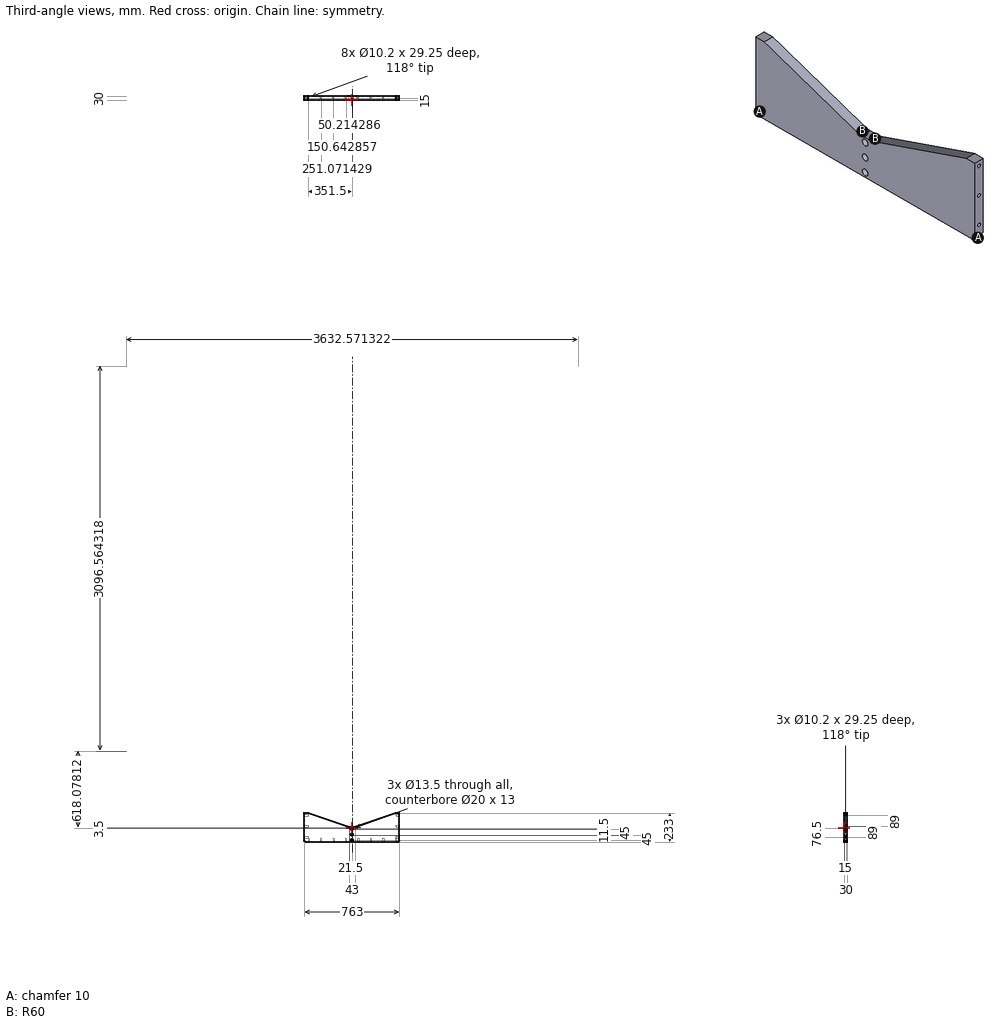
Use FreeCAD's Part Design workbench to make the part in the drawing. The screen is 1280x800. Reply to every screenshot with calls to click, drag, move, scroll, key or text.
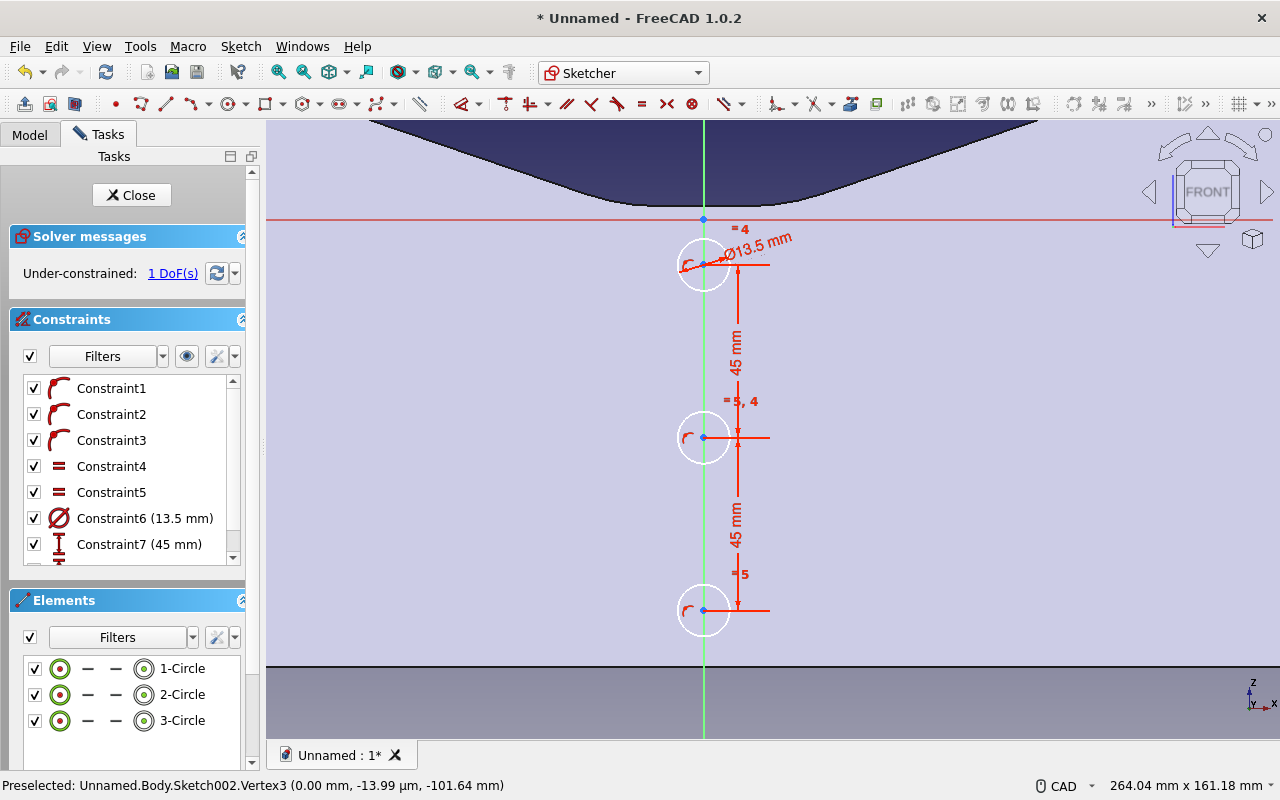
click(704, 265)
click(670, 242)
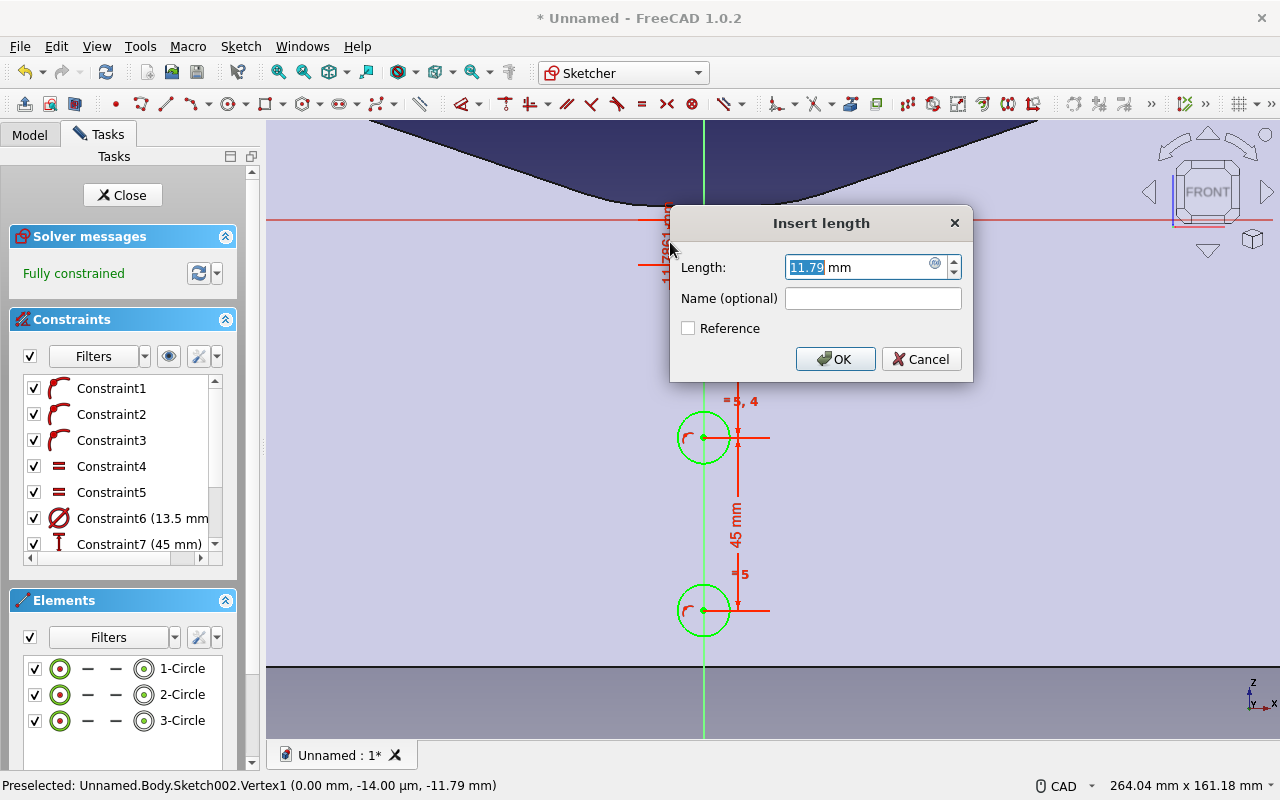
text(11.5)
key(Return)
key(Escape)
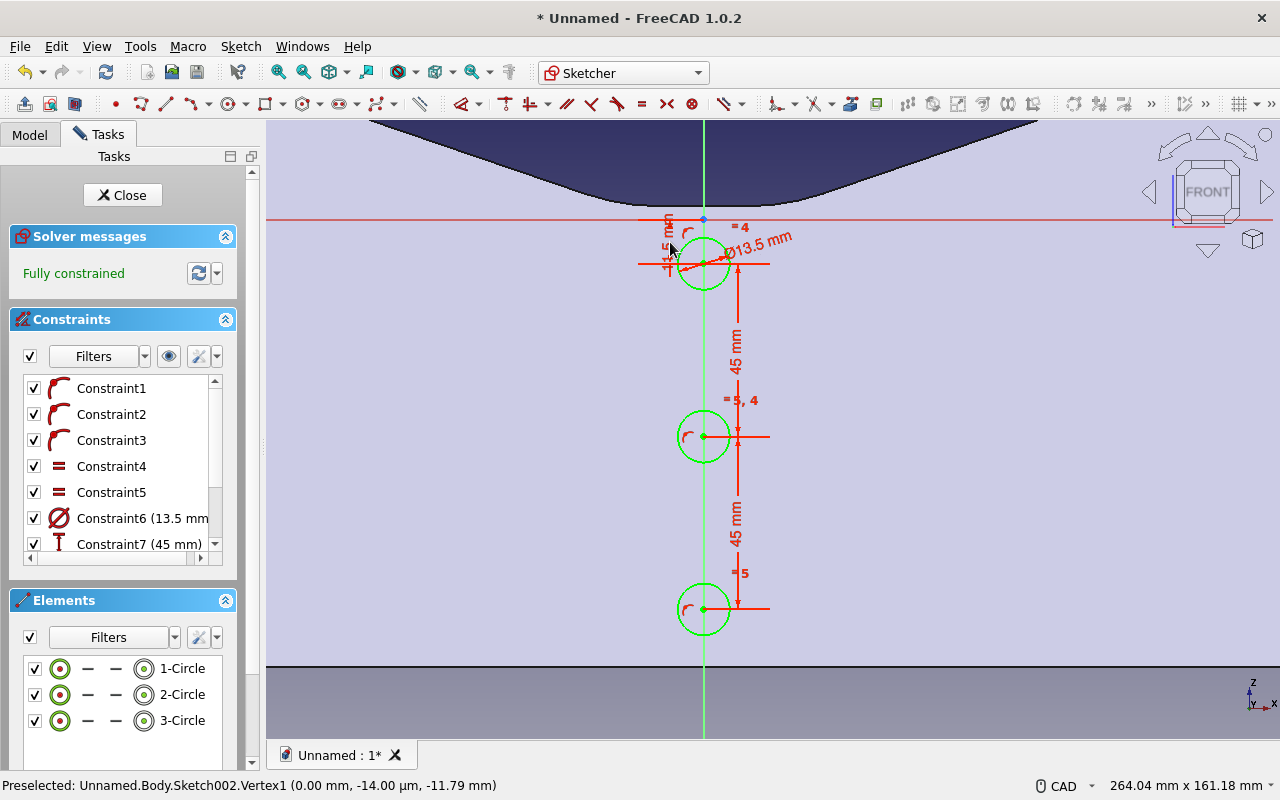
click(123, 195)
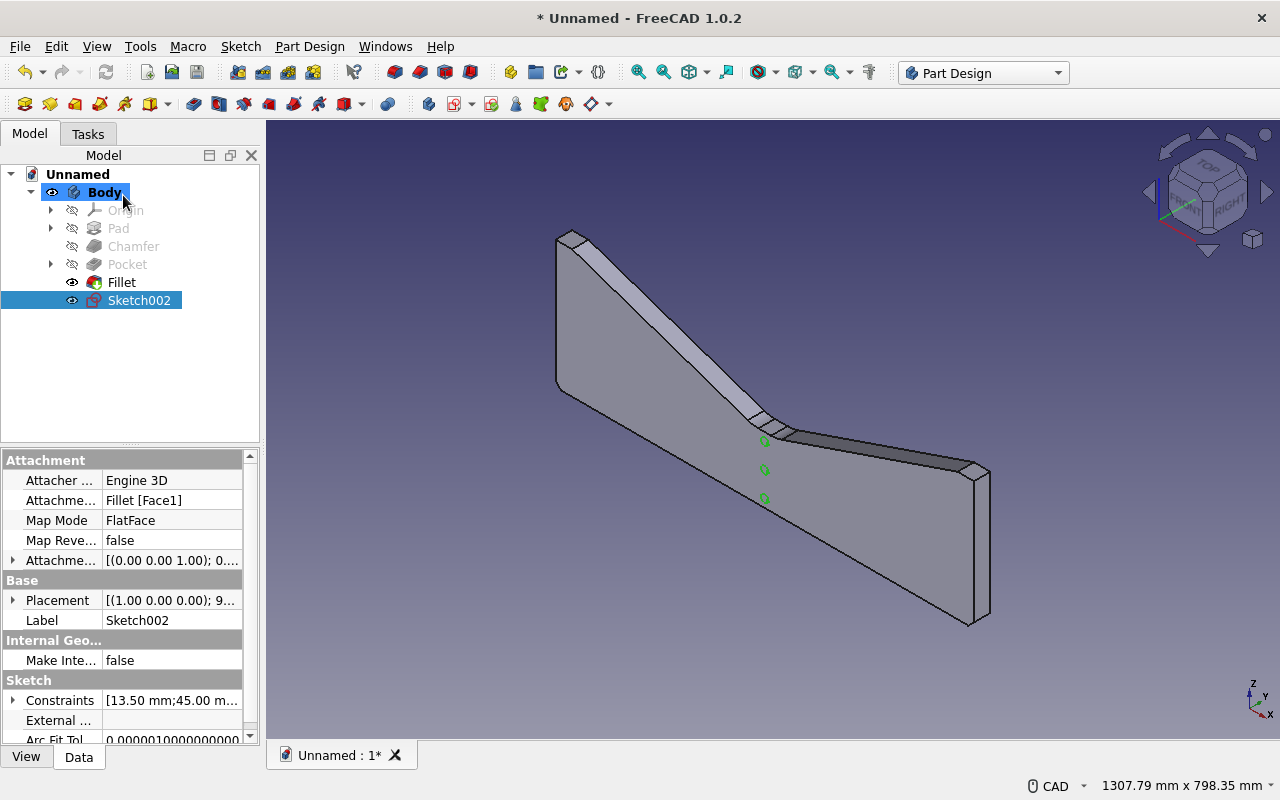
click(219, 104)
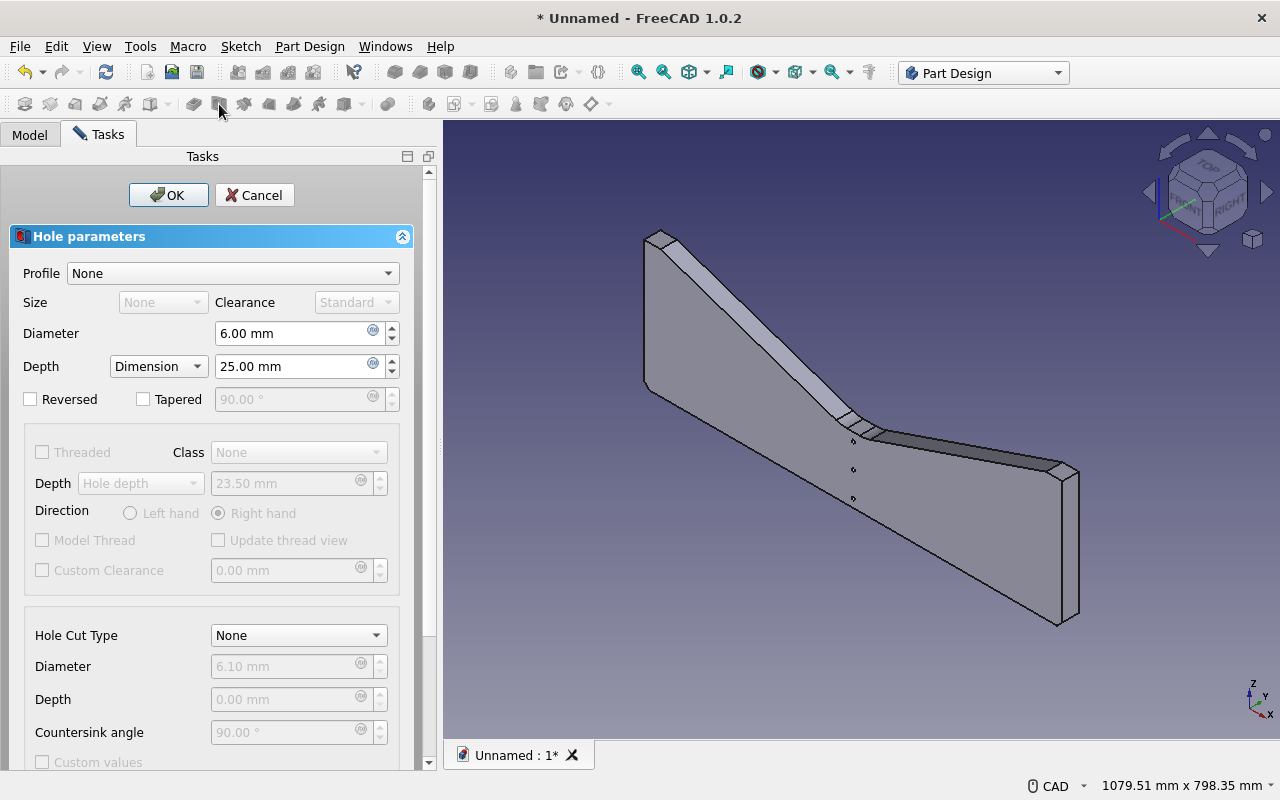
triple_click(300, 334)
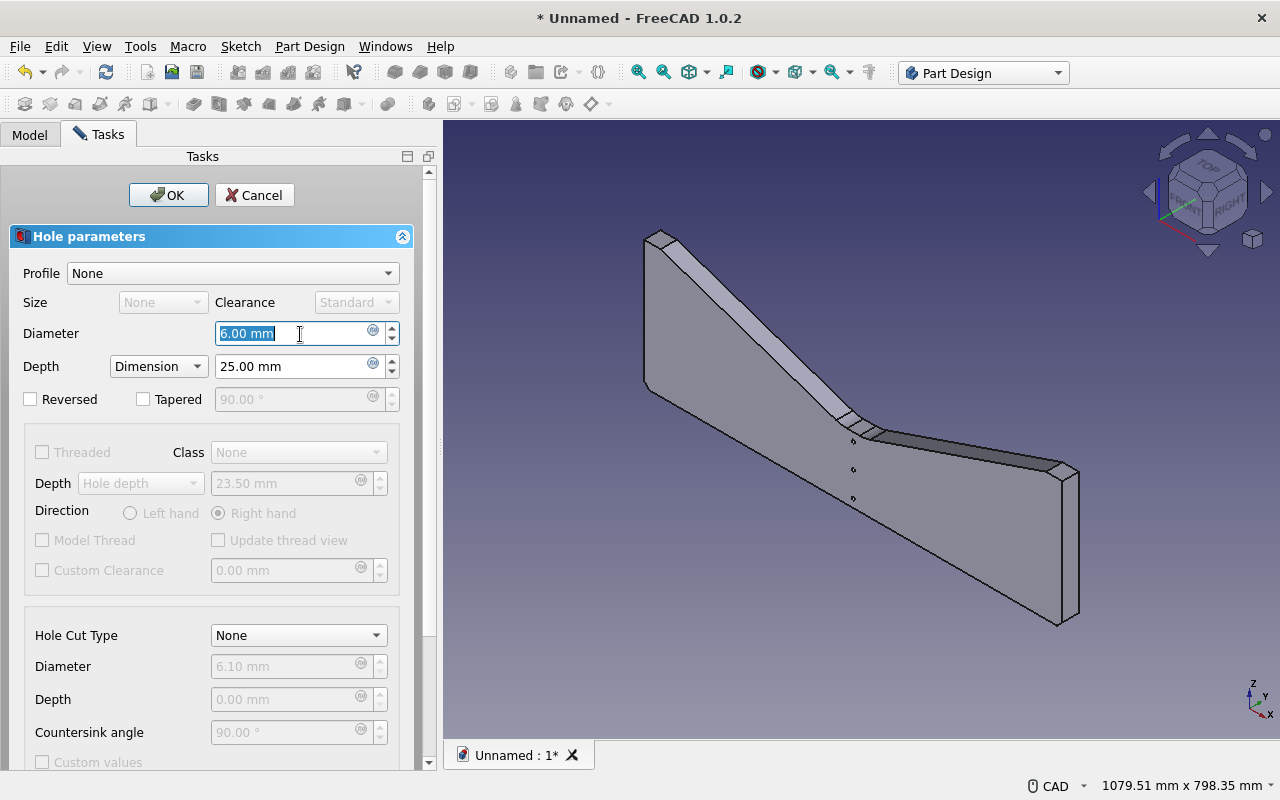
text(13.5)
key(Tab)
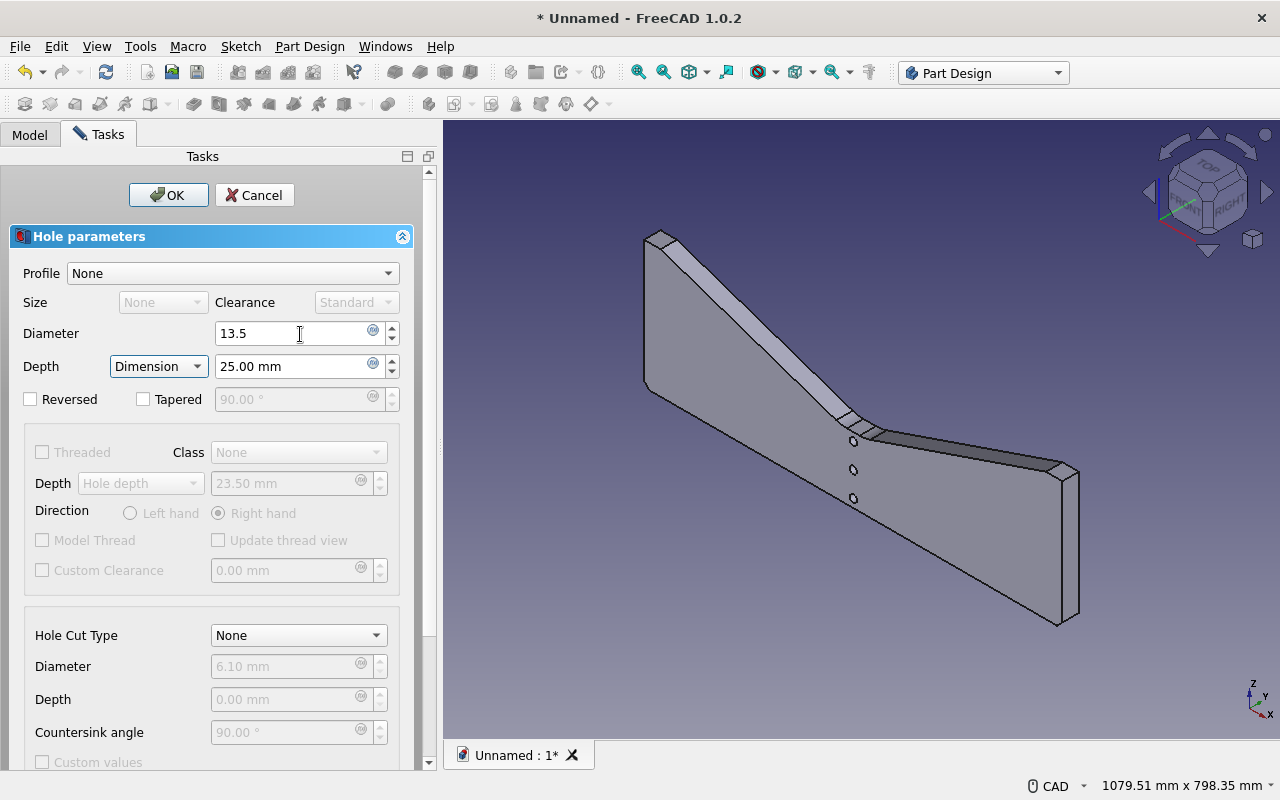
click(160, 366)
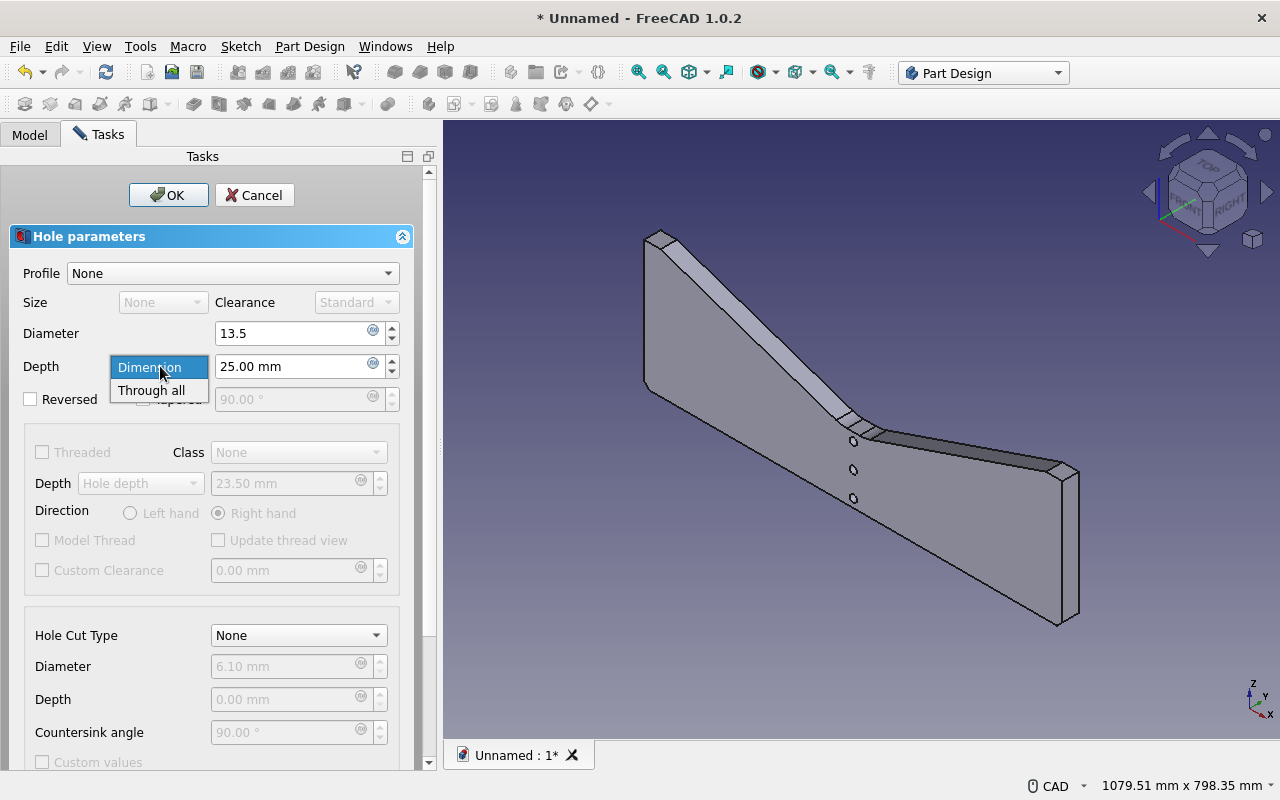
click(158, 390)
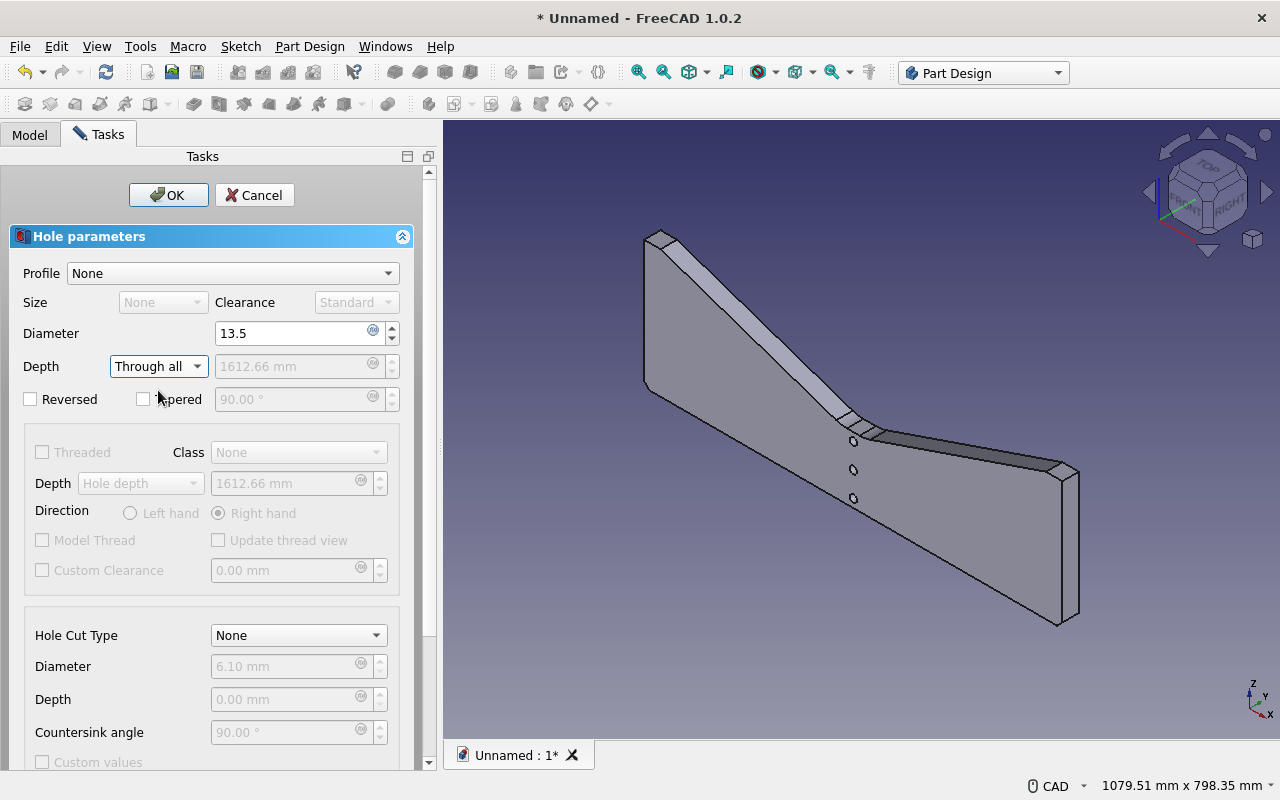
click(300, 636)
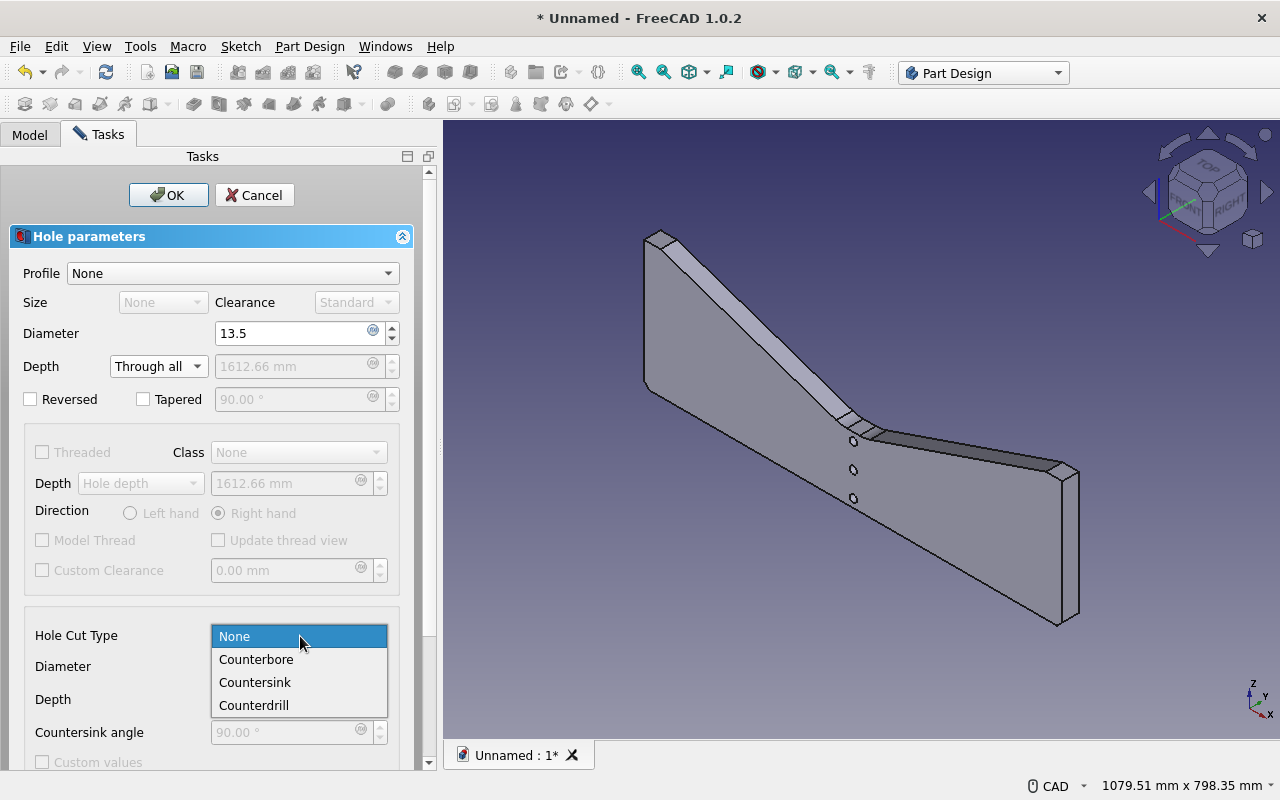
click(298, 660)